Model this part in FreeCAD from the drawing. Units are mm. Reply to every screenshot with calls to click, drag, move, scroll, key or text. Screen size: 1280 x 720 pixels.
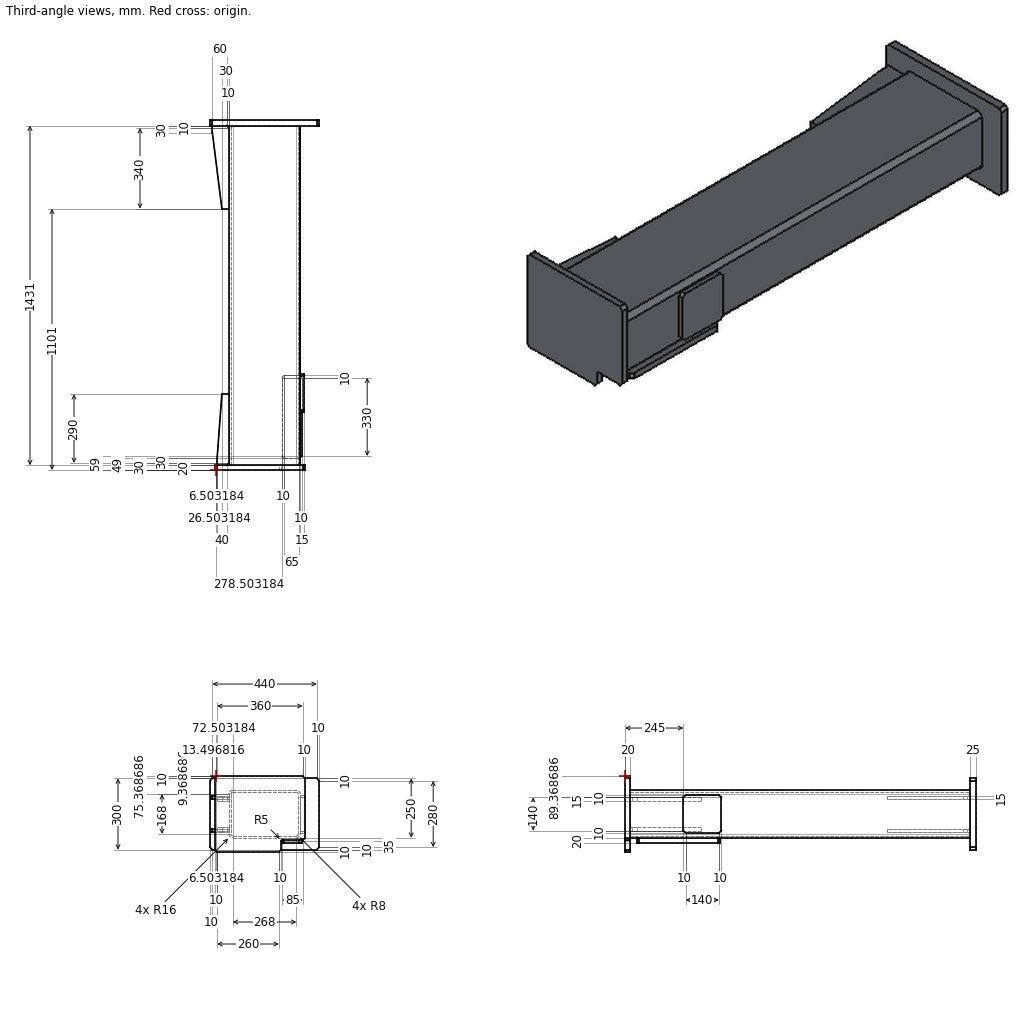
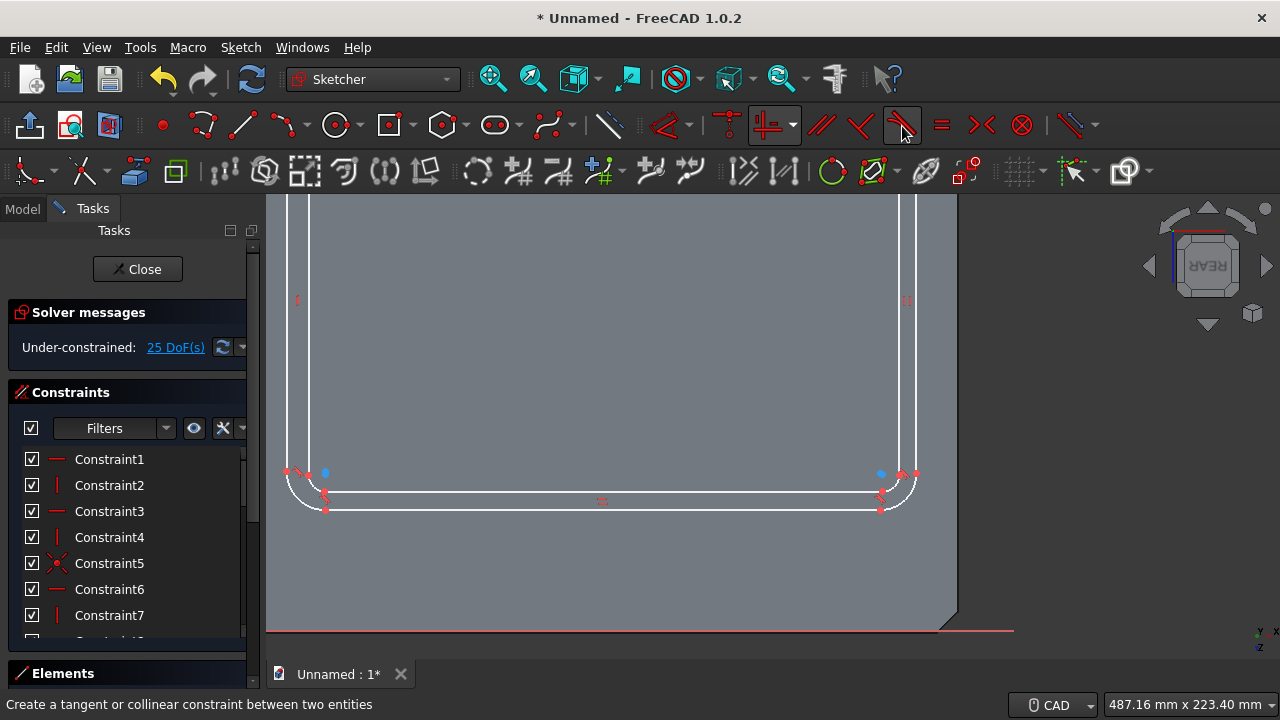
click(916, 370)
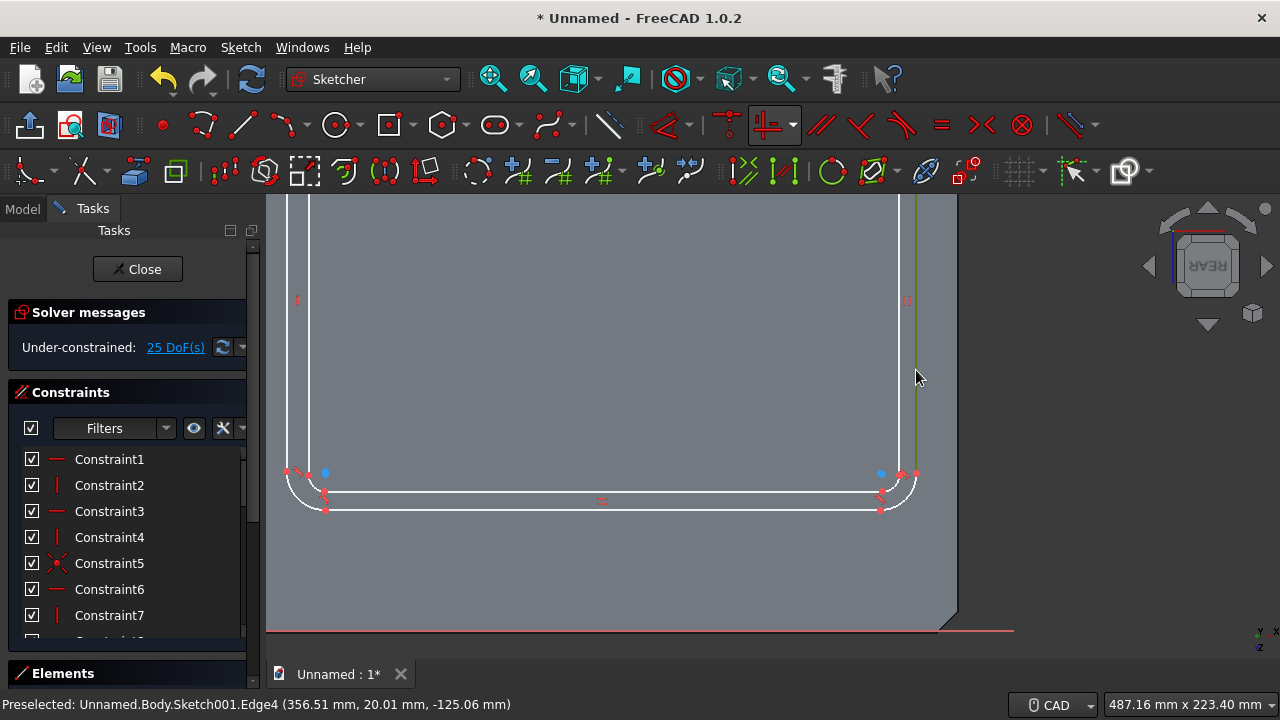
scroll(898, 506, down, 3)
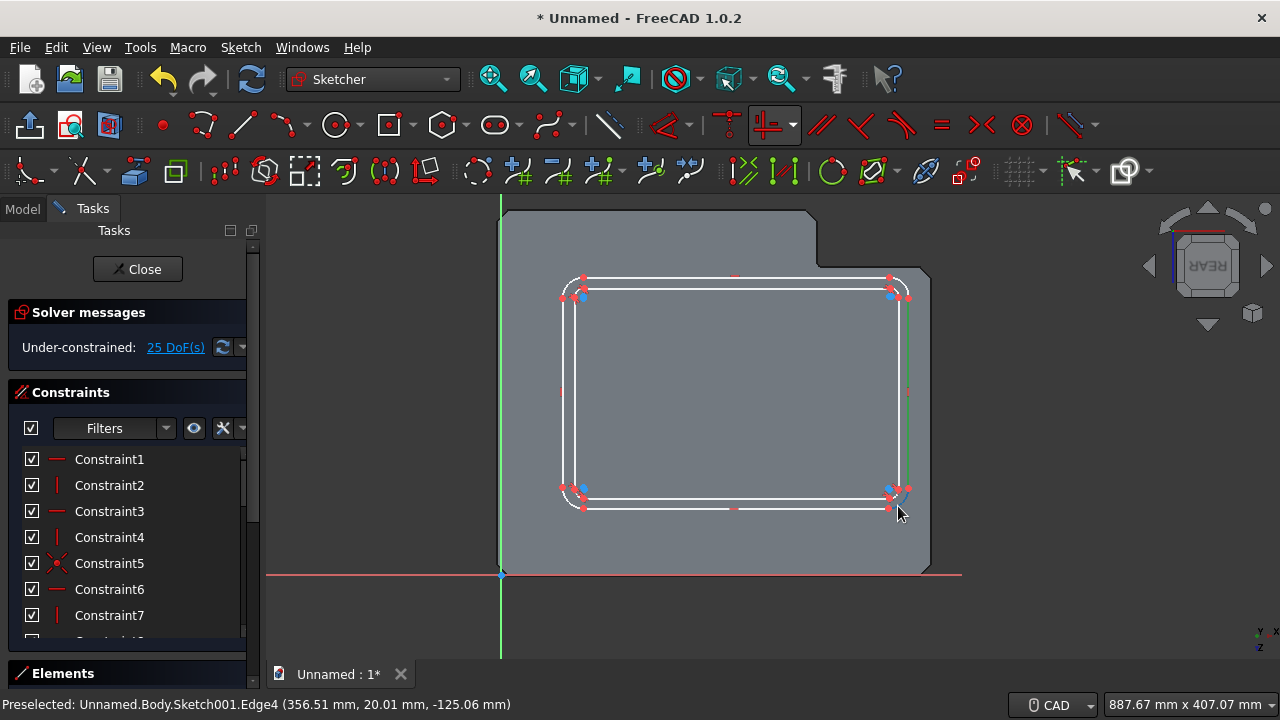
scroll(907, 289, up, 3)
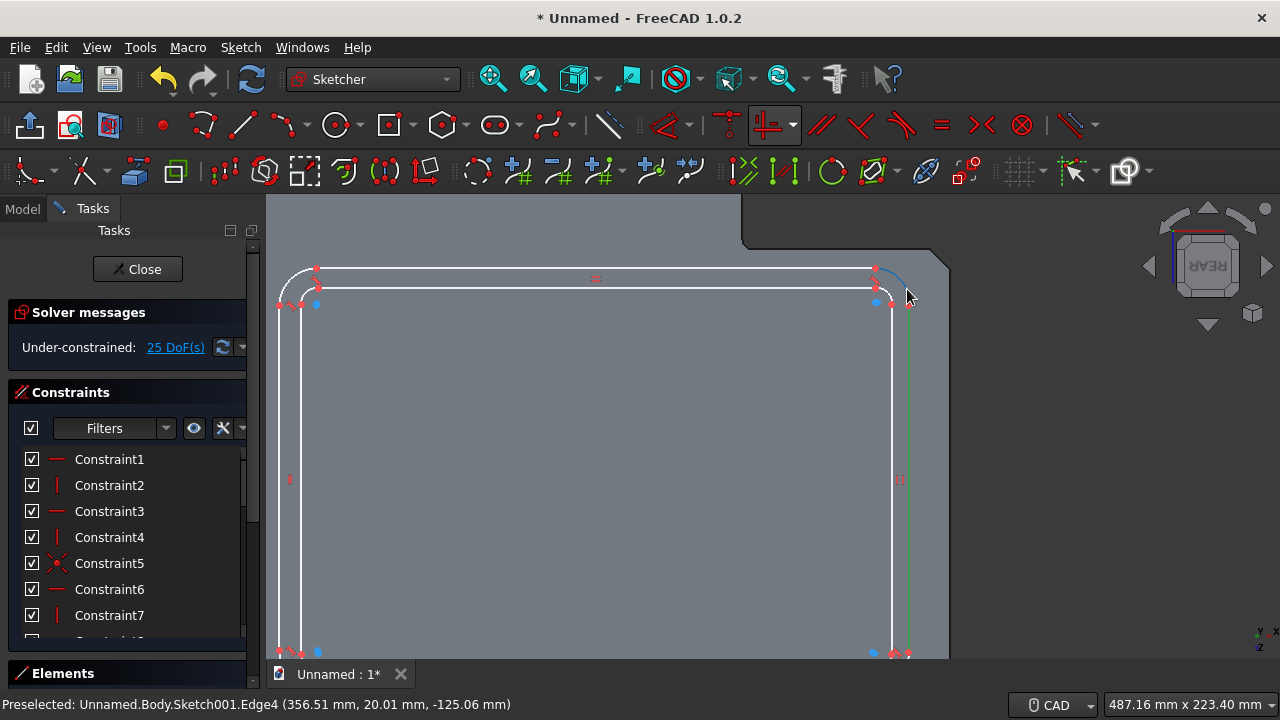
click(907, 289)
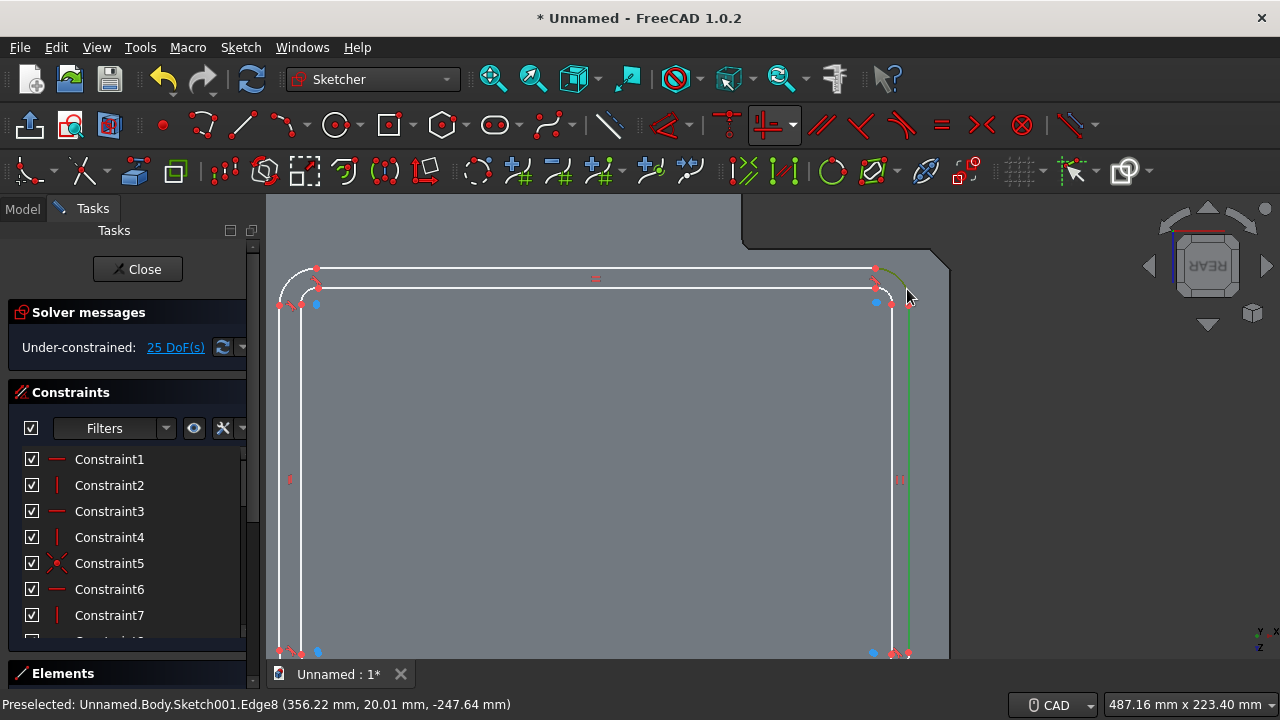
click(902, 126)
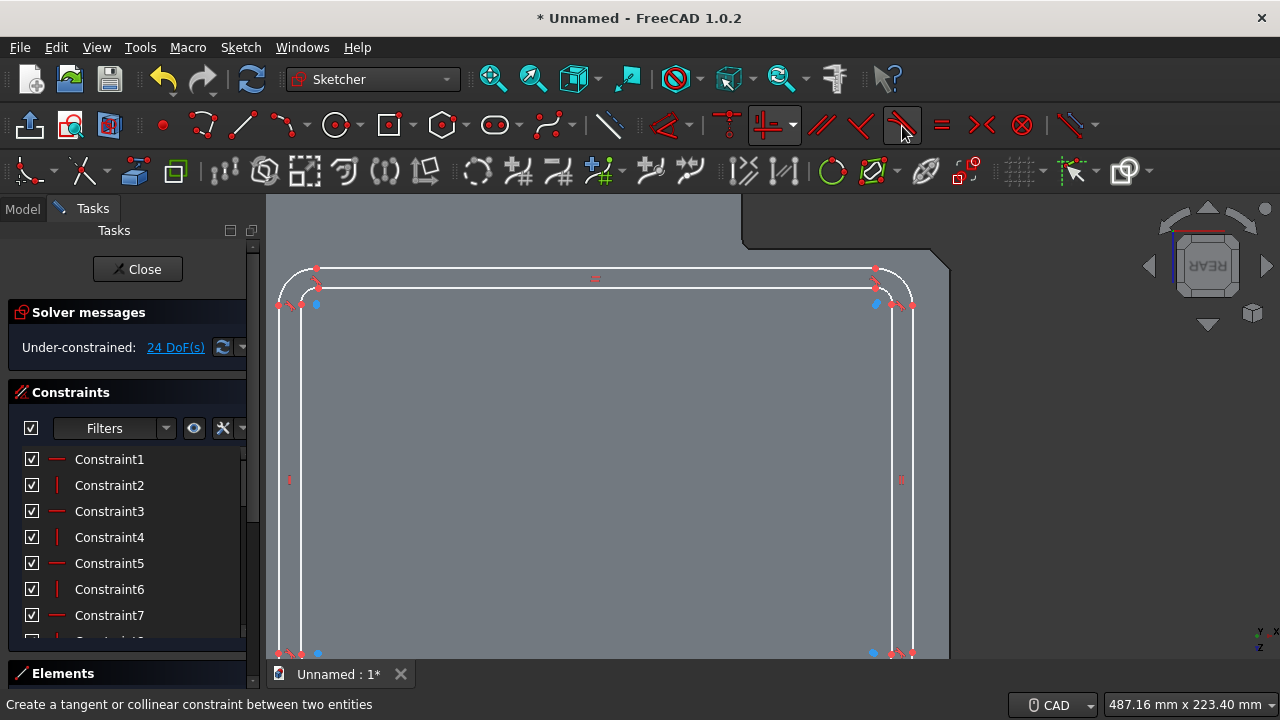
click(485, 288)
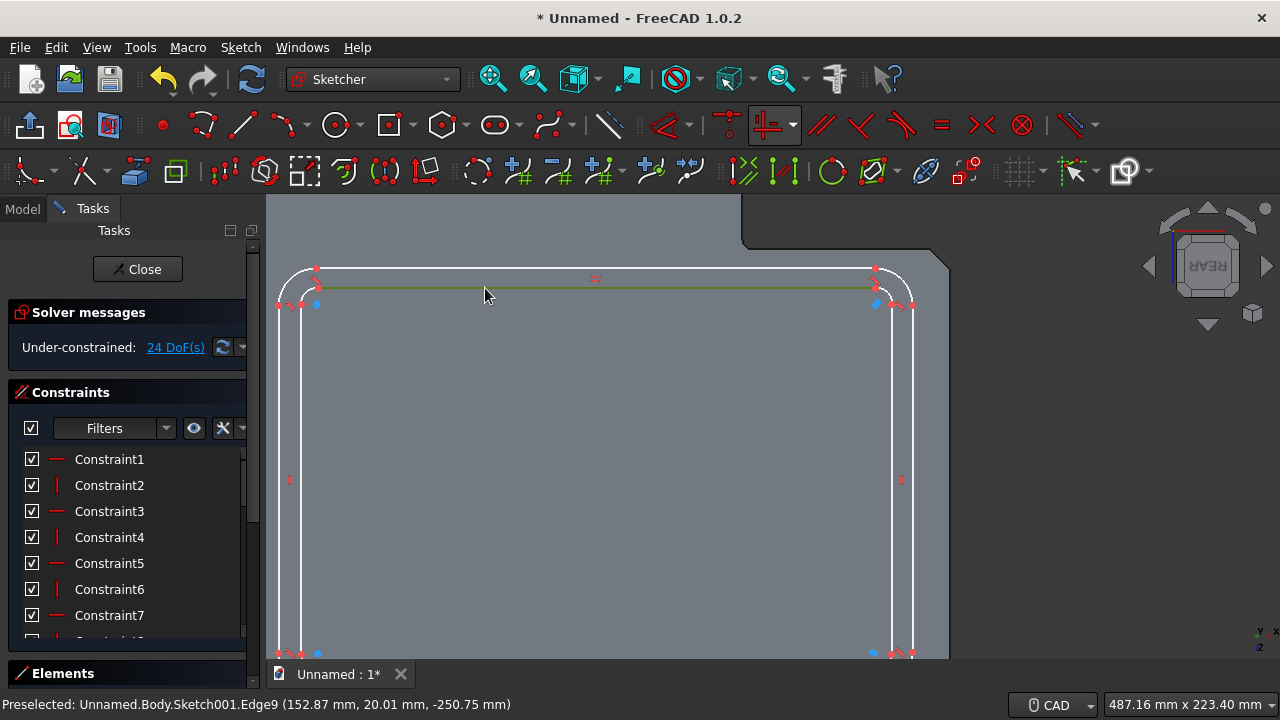
click(888, 292)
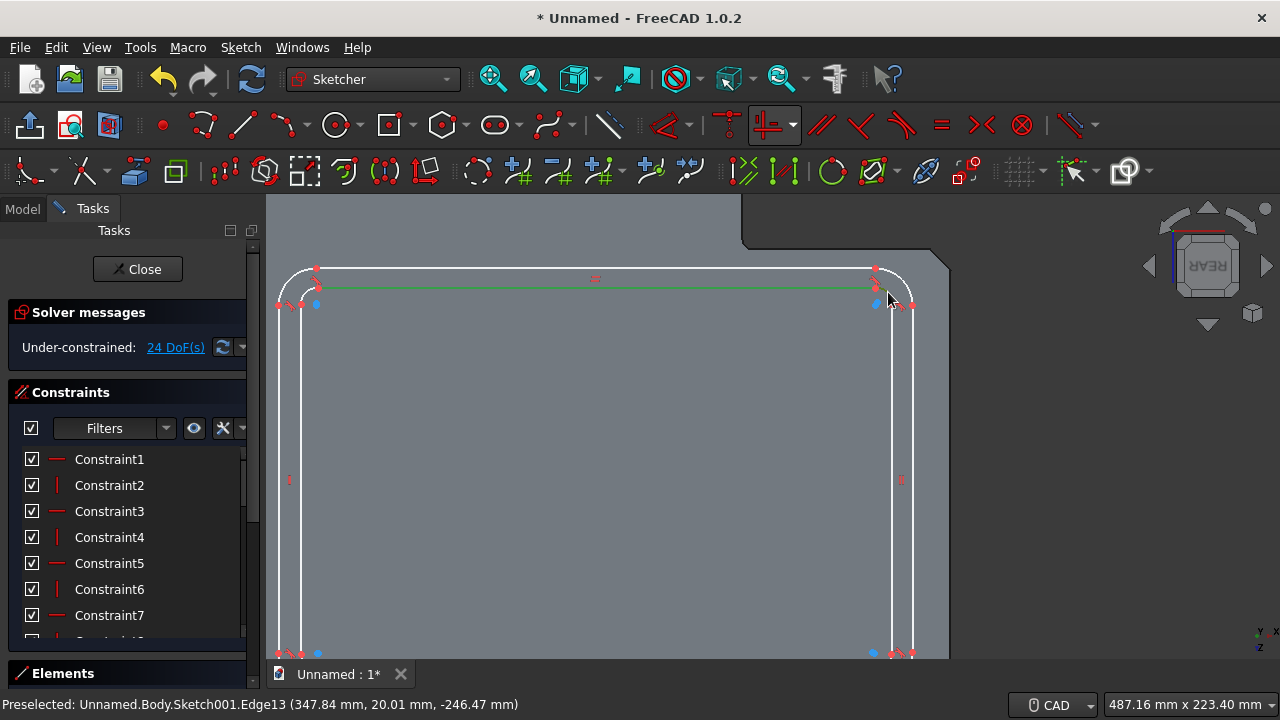
click(902, 126)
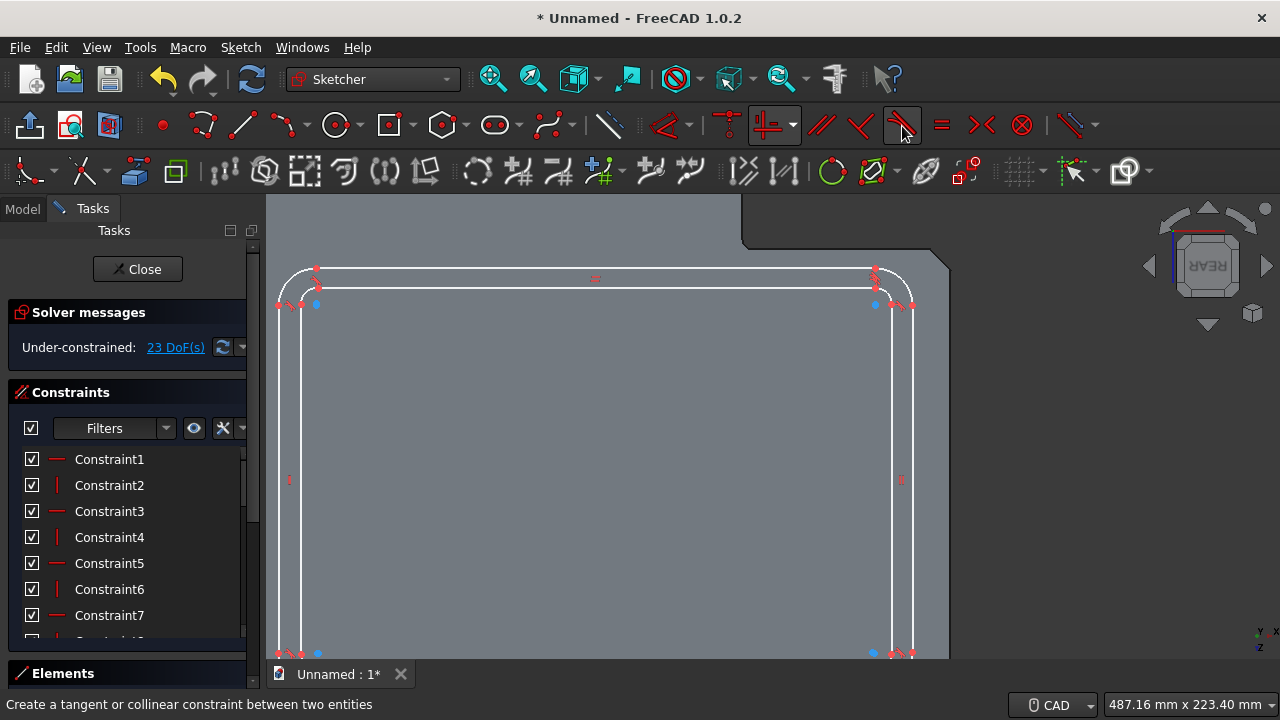
click(485, 288)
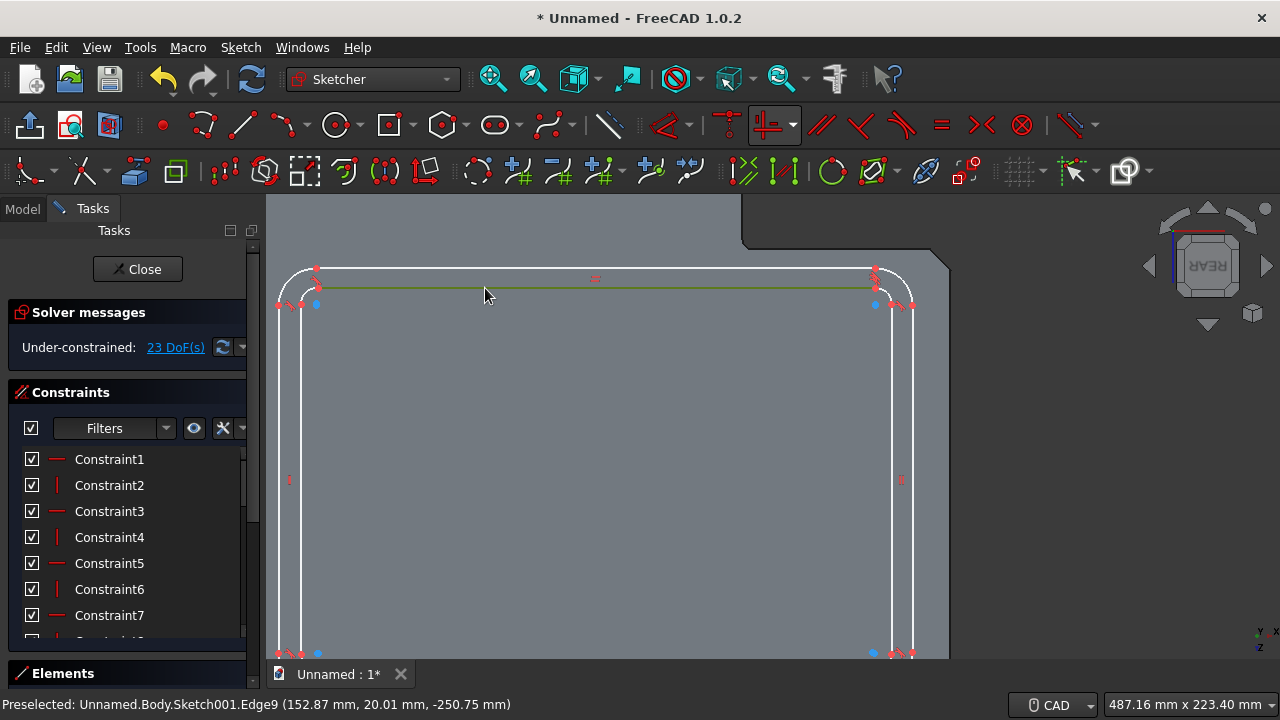
click(306, 292)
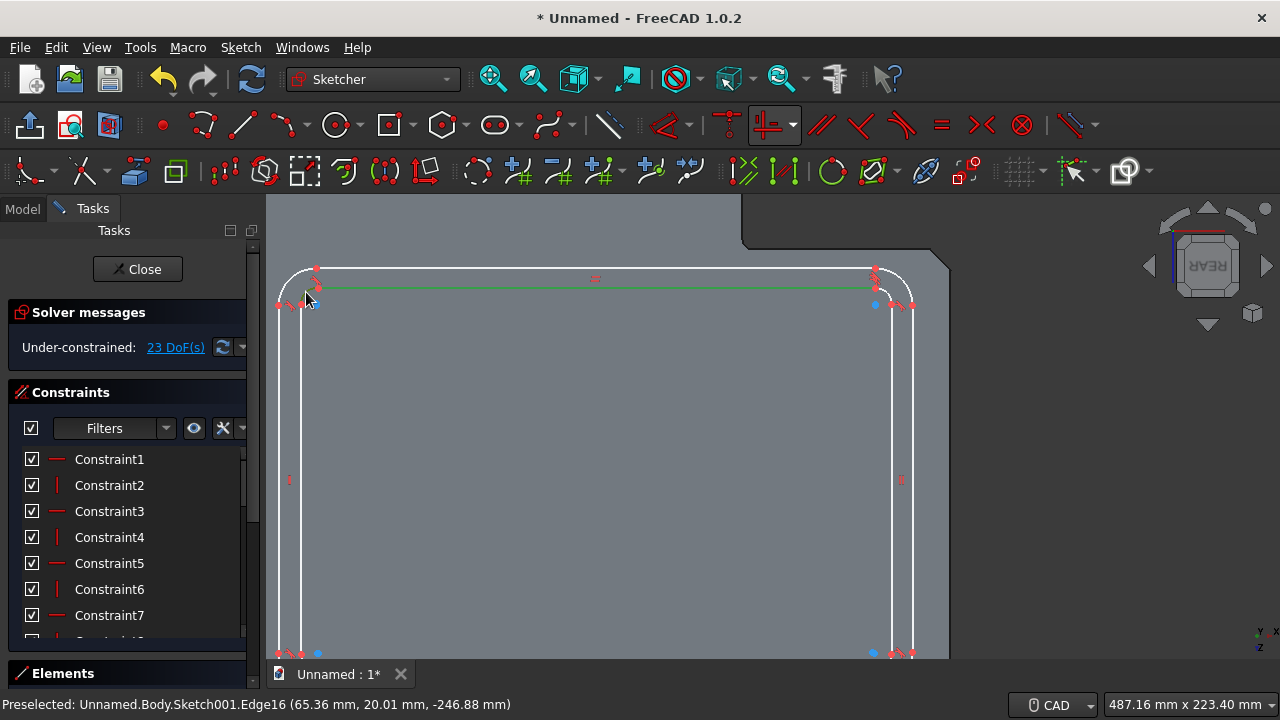
key(t)